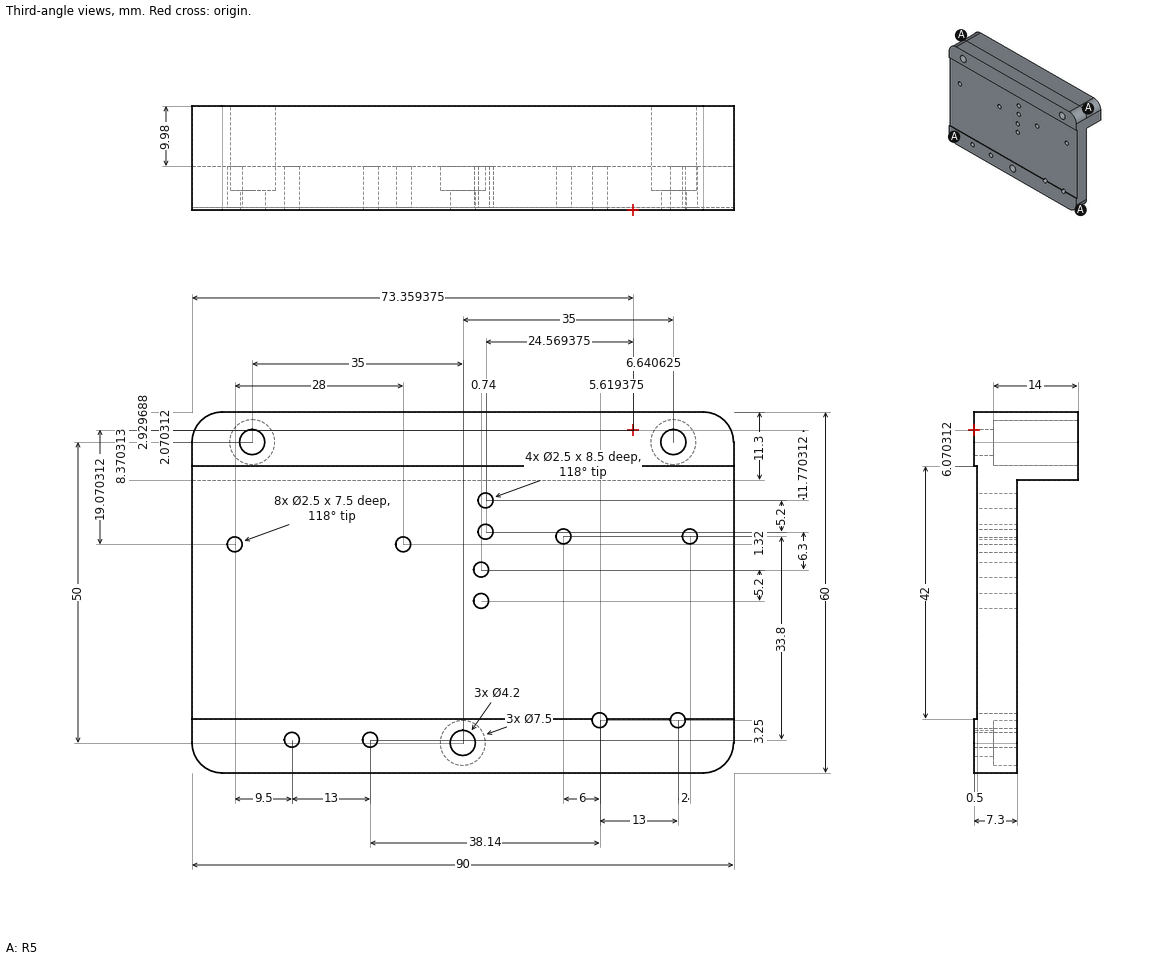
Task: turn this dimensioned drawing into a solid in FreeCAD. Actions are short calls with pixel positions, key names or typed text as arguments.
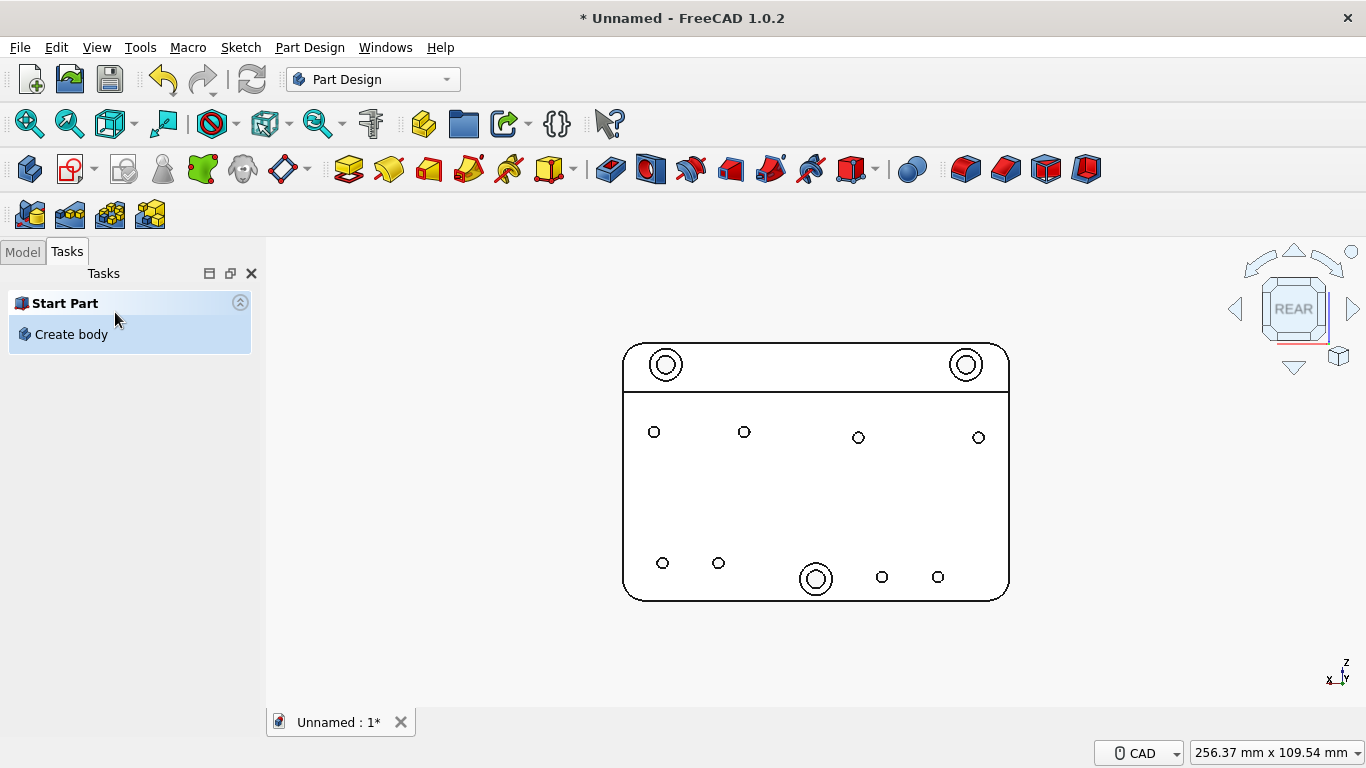
click(926, 495)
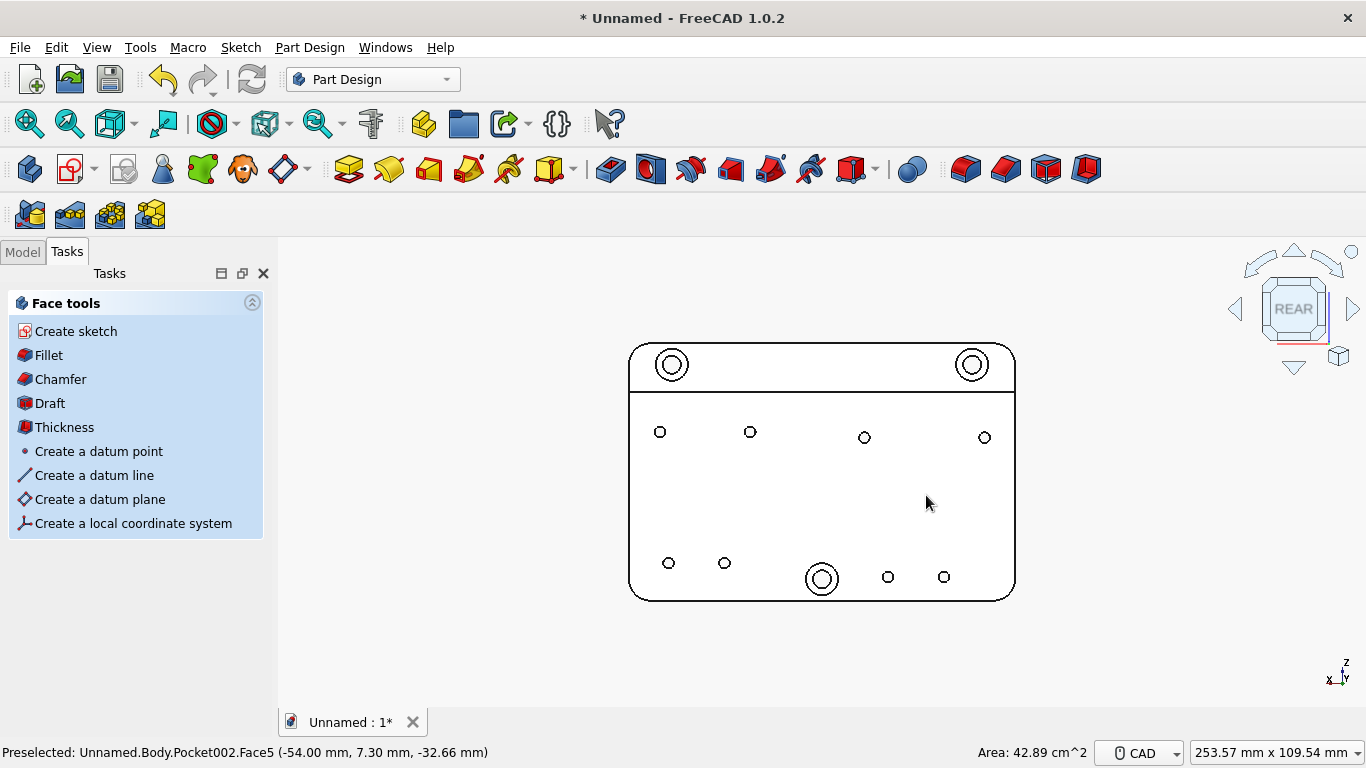
click(70, 170)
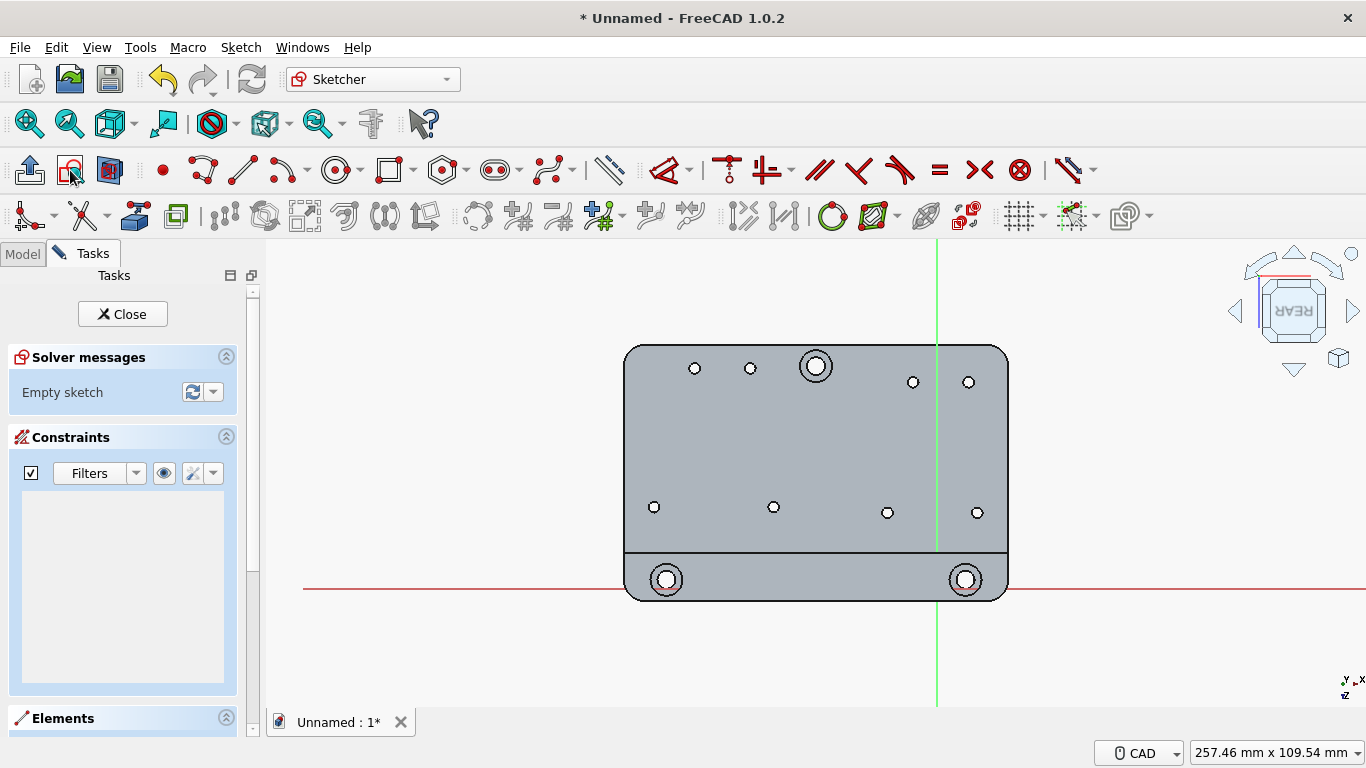
click(110, 170)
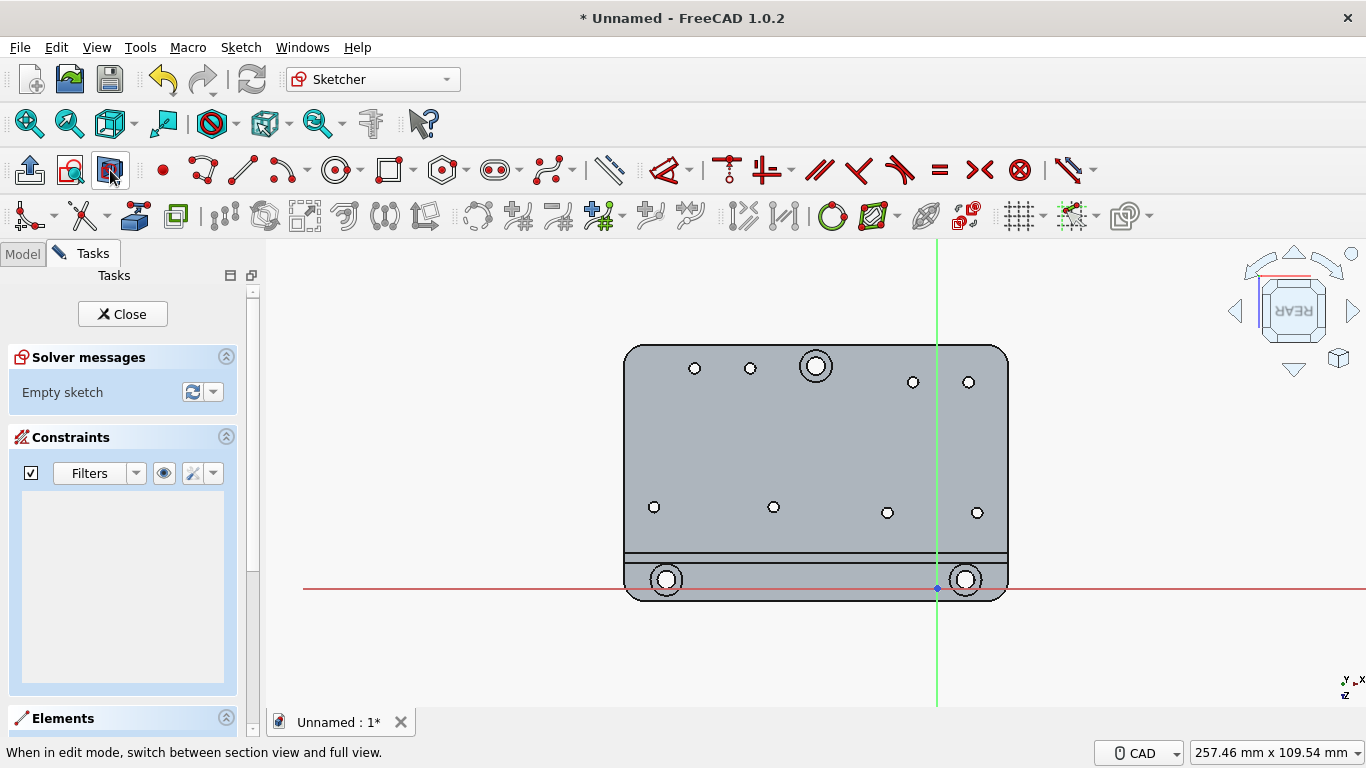
scroll(989, 568, up, 4)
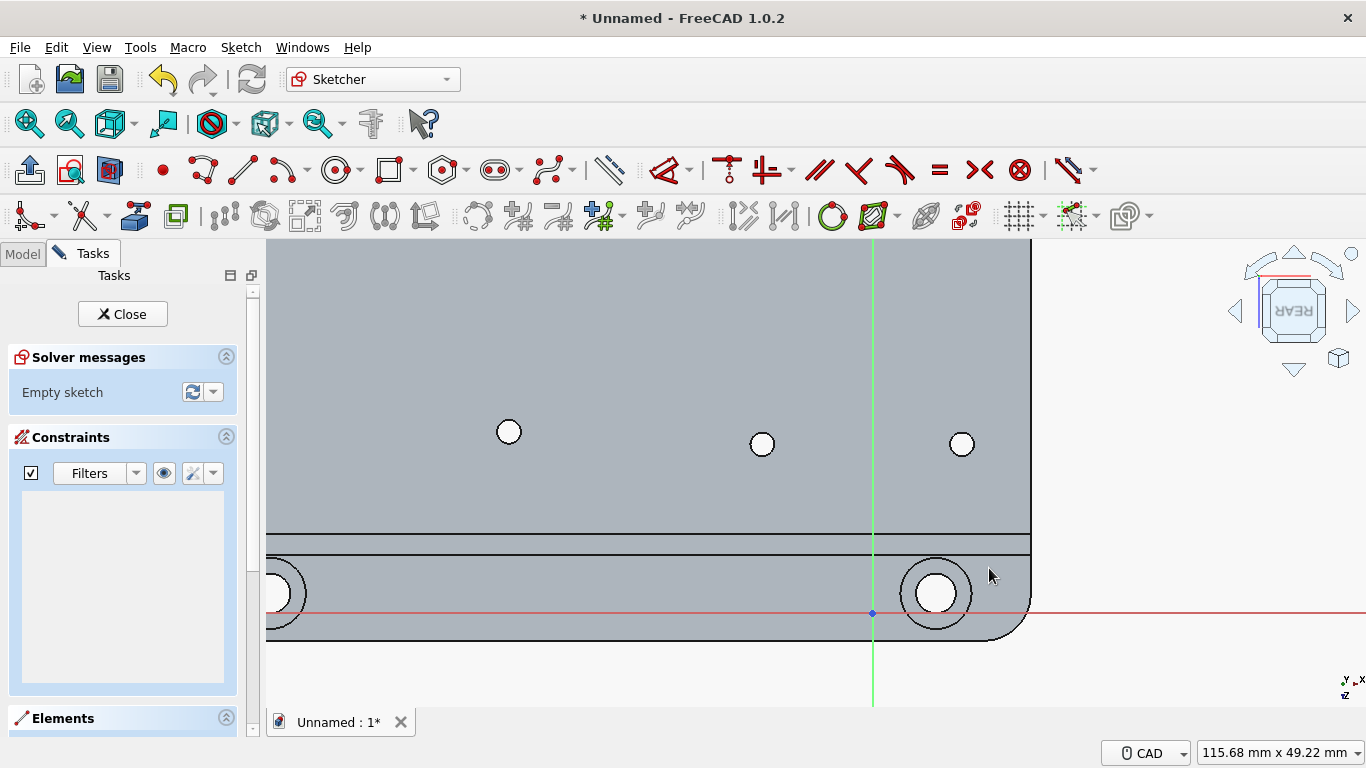
click(336, 170)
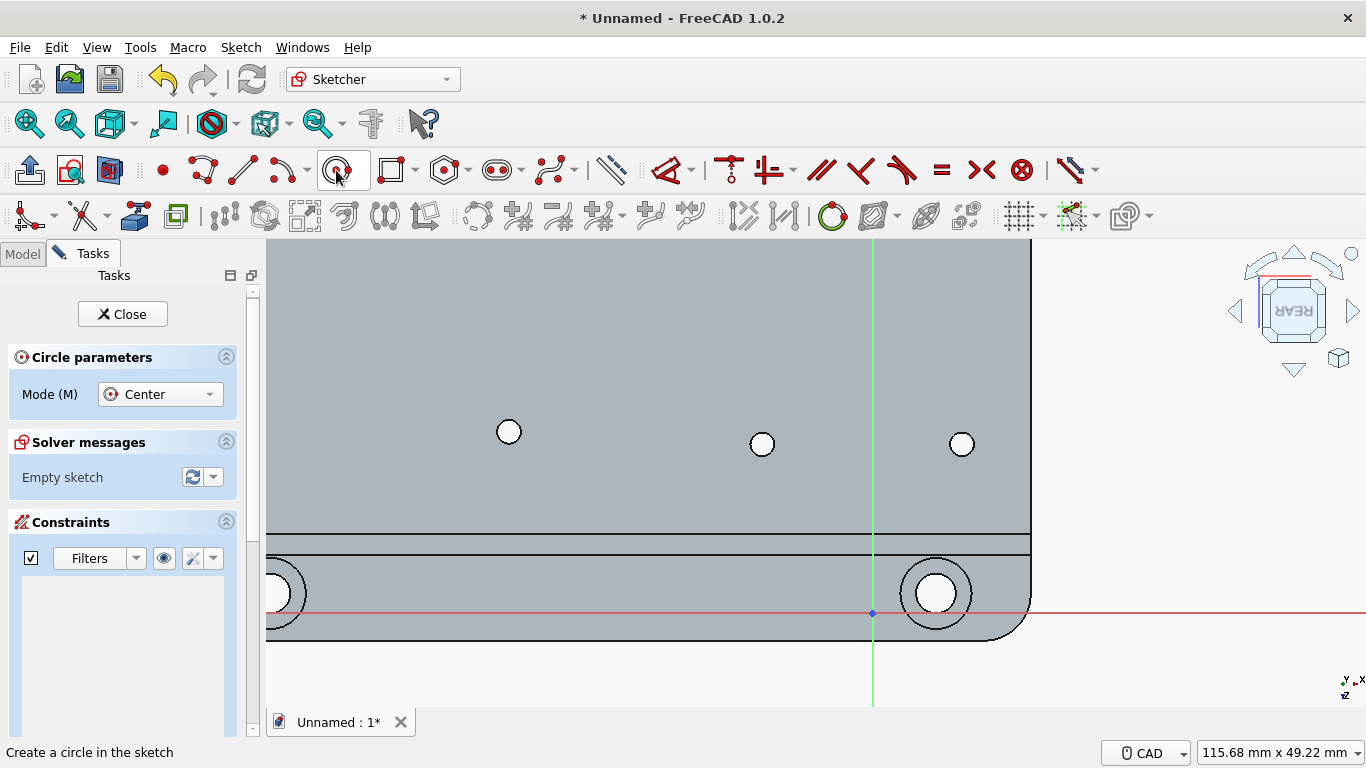
scroll(639, 501, up, 4)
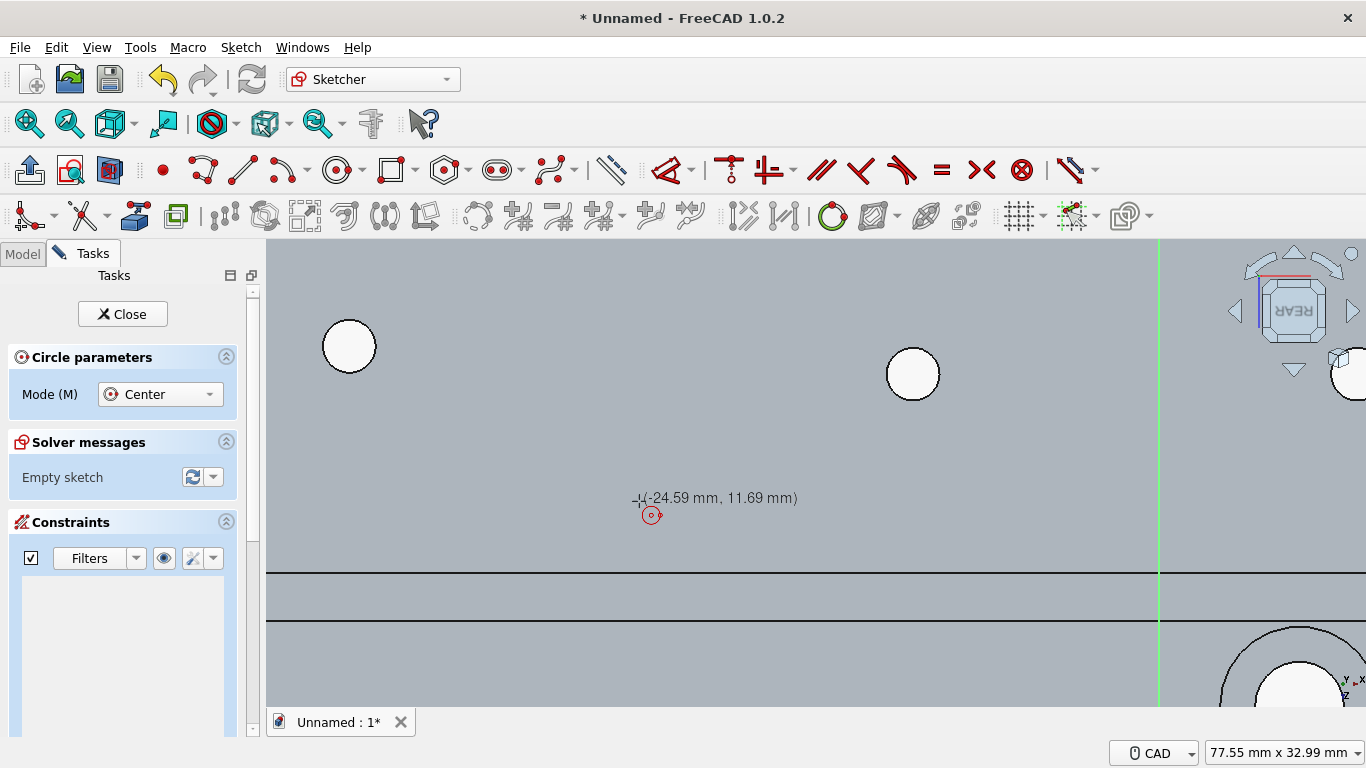
click(639, 501)
move(658, 482)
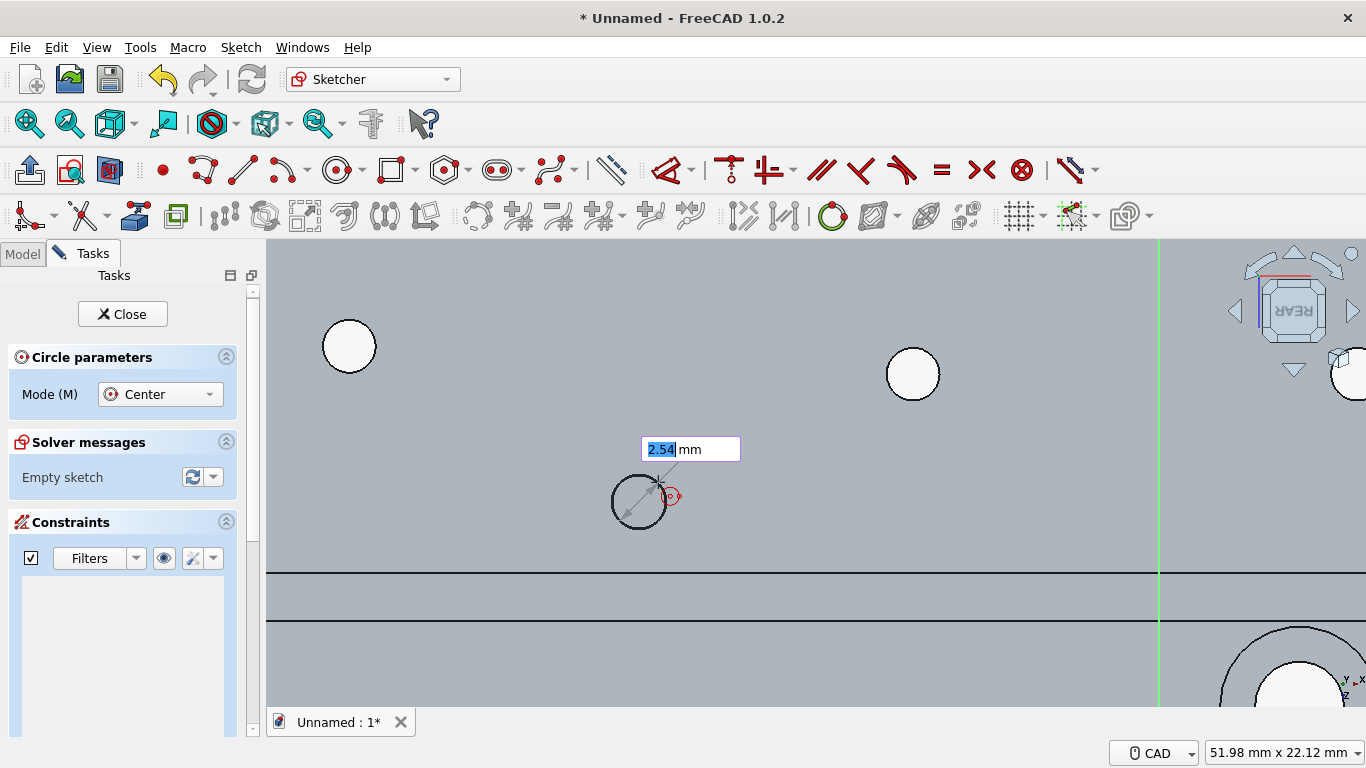
text(2.5)
key(Return)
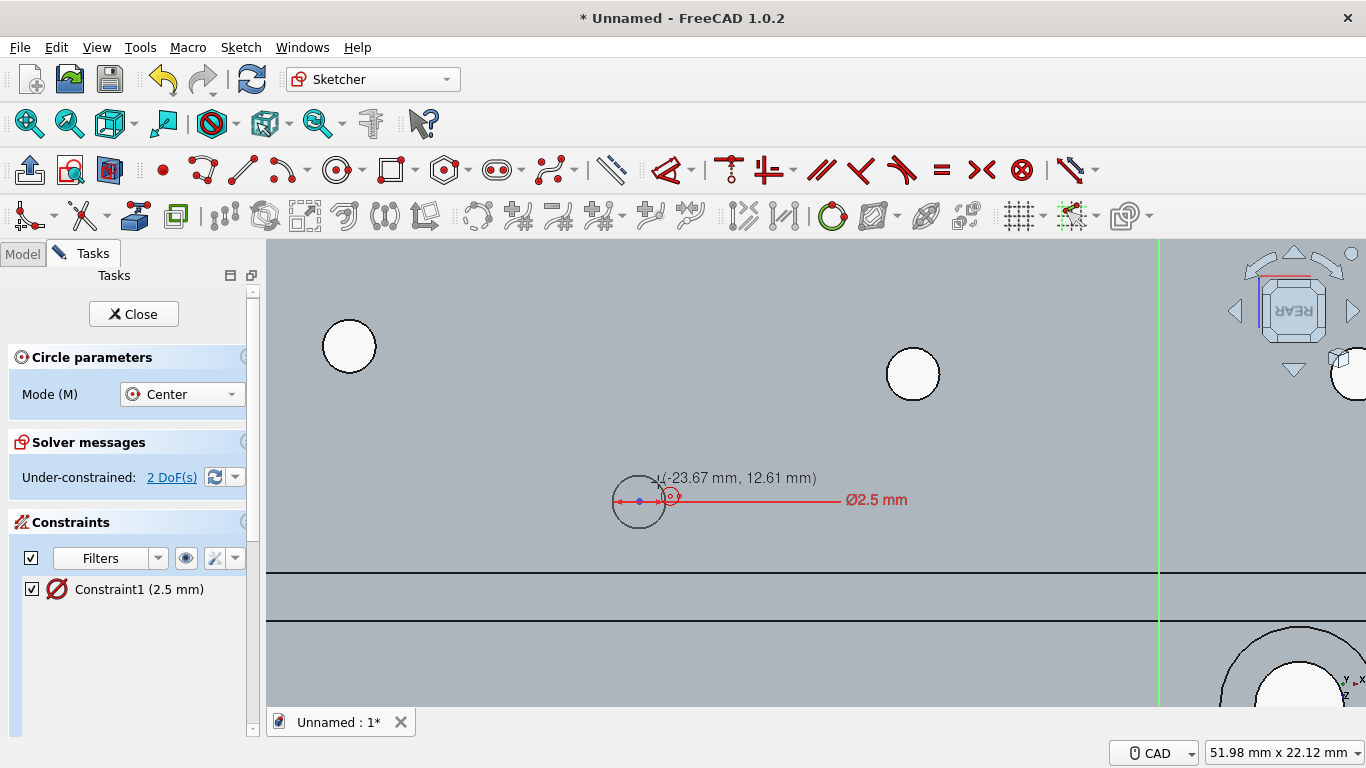
click(639, 391)
move(658, 372)